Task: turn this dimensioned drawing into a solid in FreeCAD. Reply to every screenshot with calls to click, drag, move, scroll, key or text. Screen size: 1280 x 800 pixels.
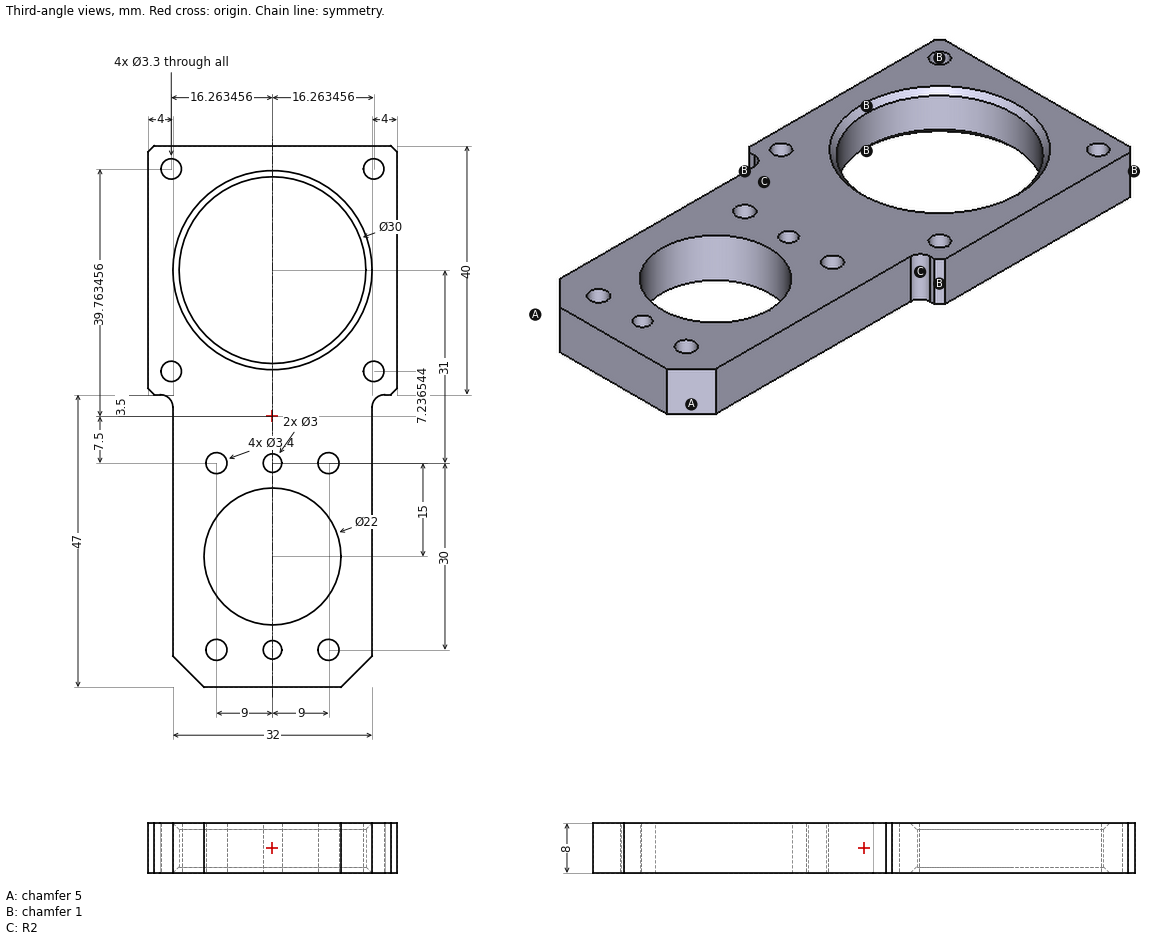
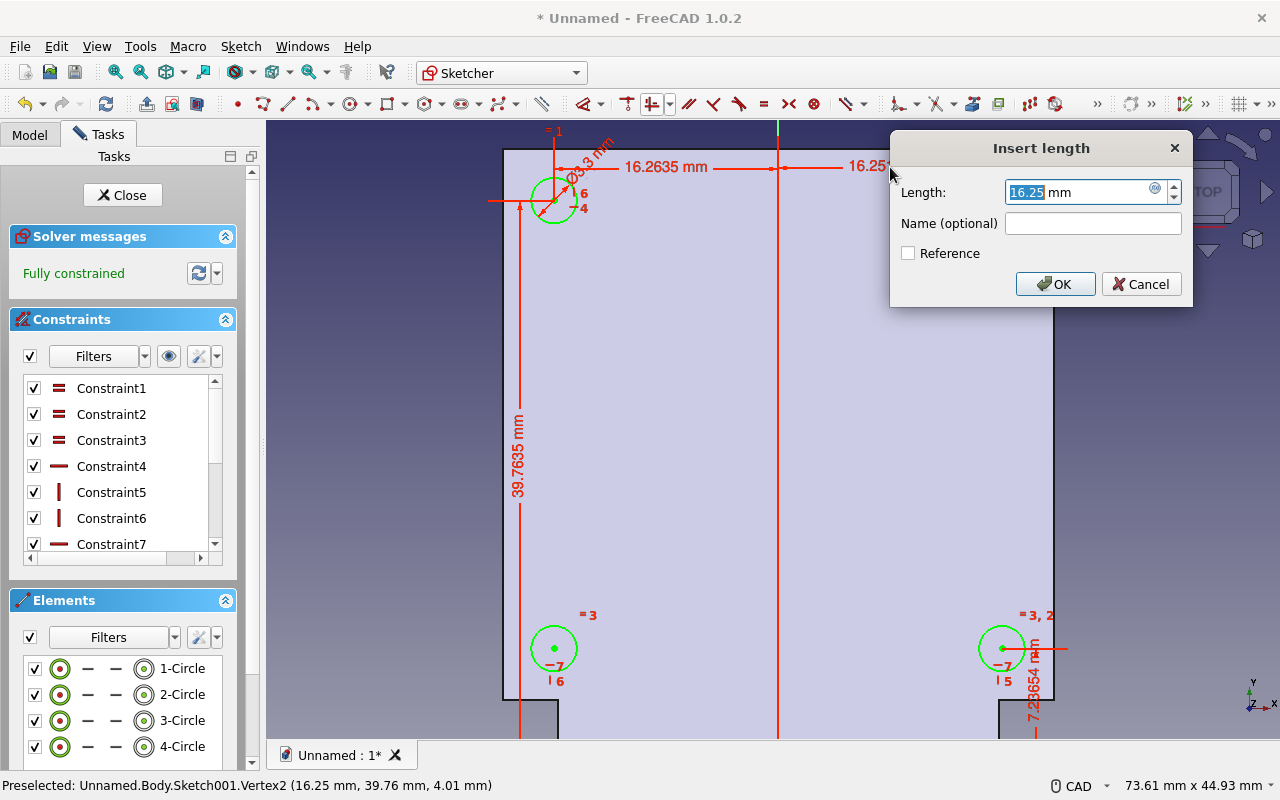
text(16.263456)
key(Return)
key(Escape)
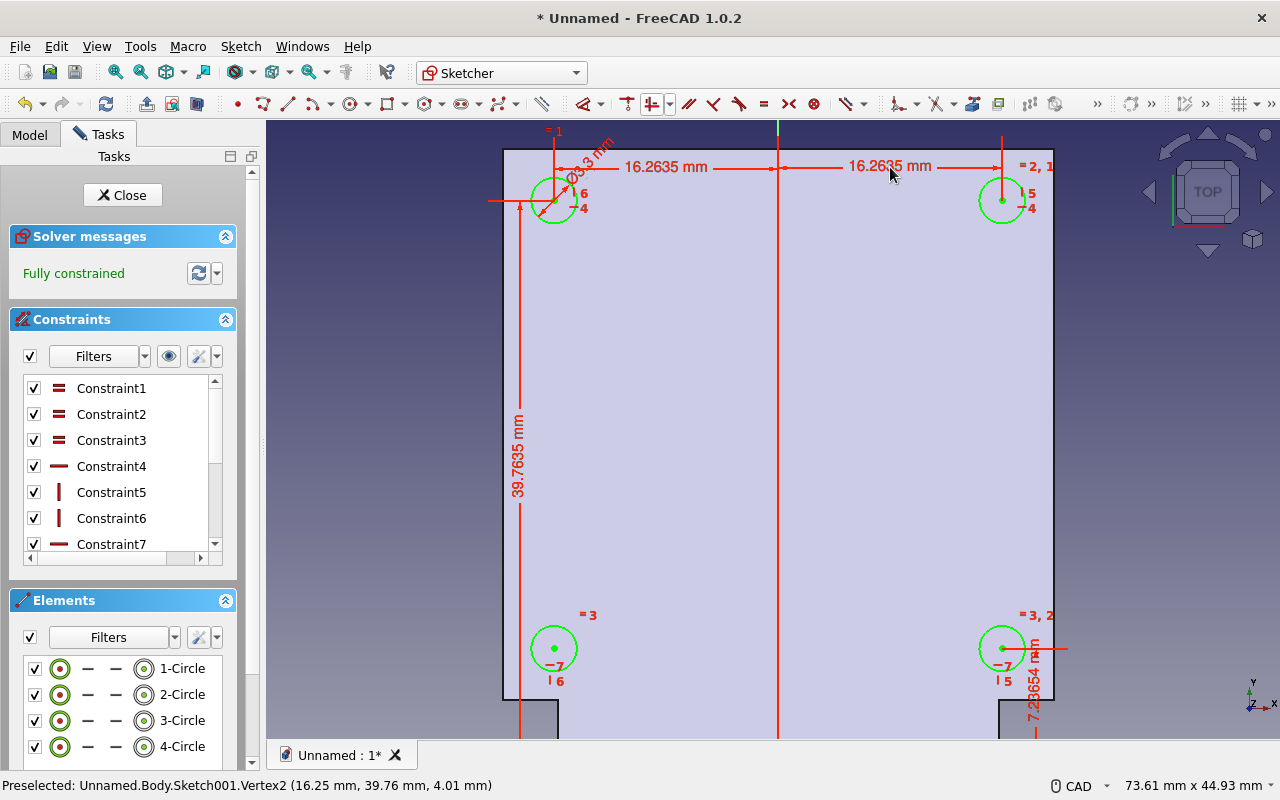
click(123, 195)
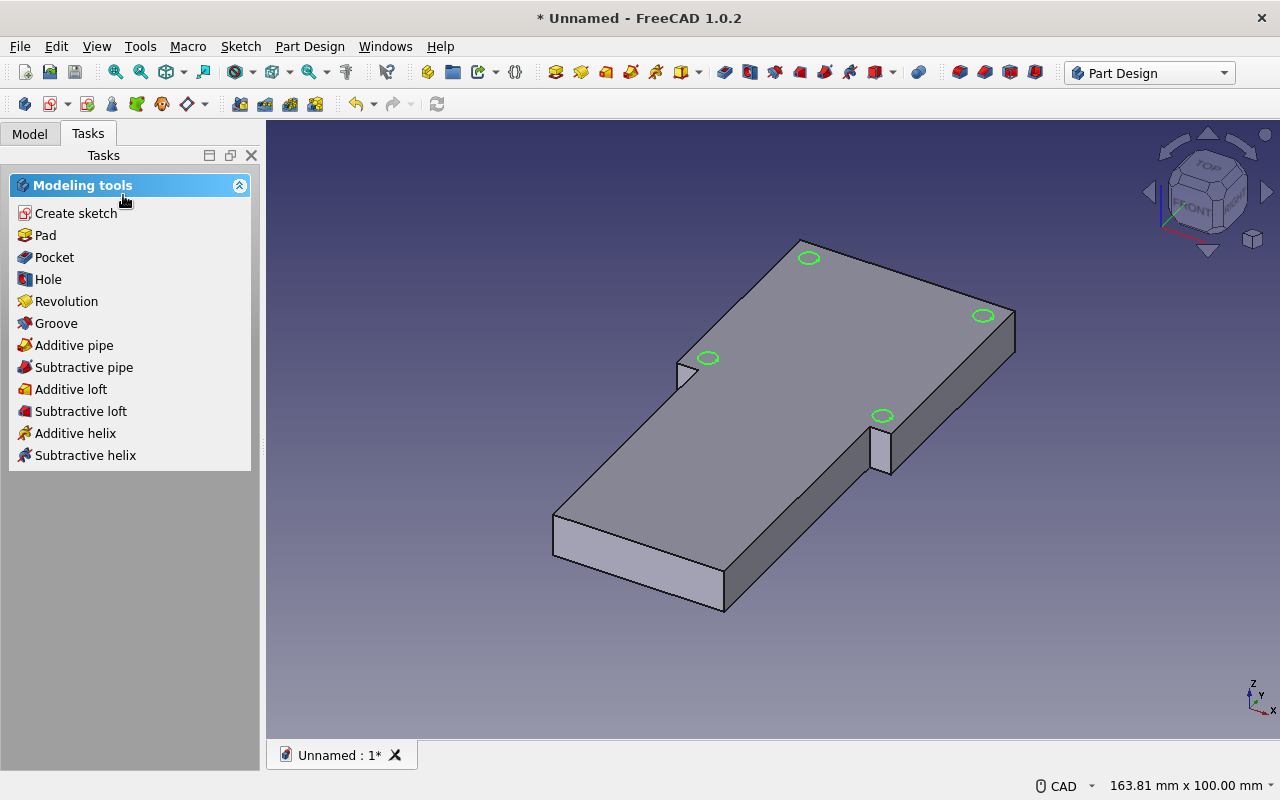
click(750, 72)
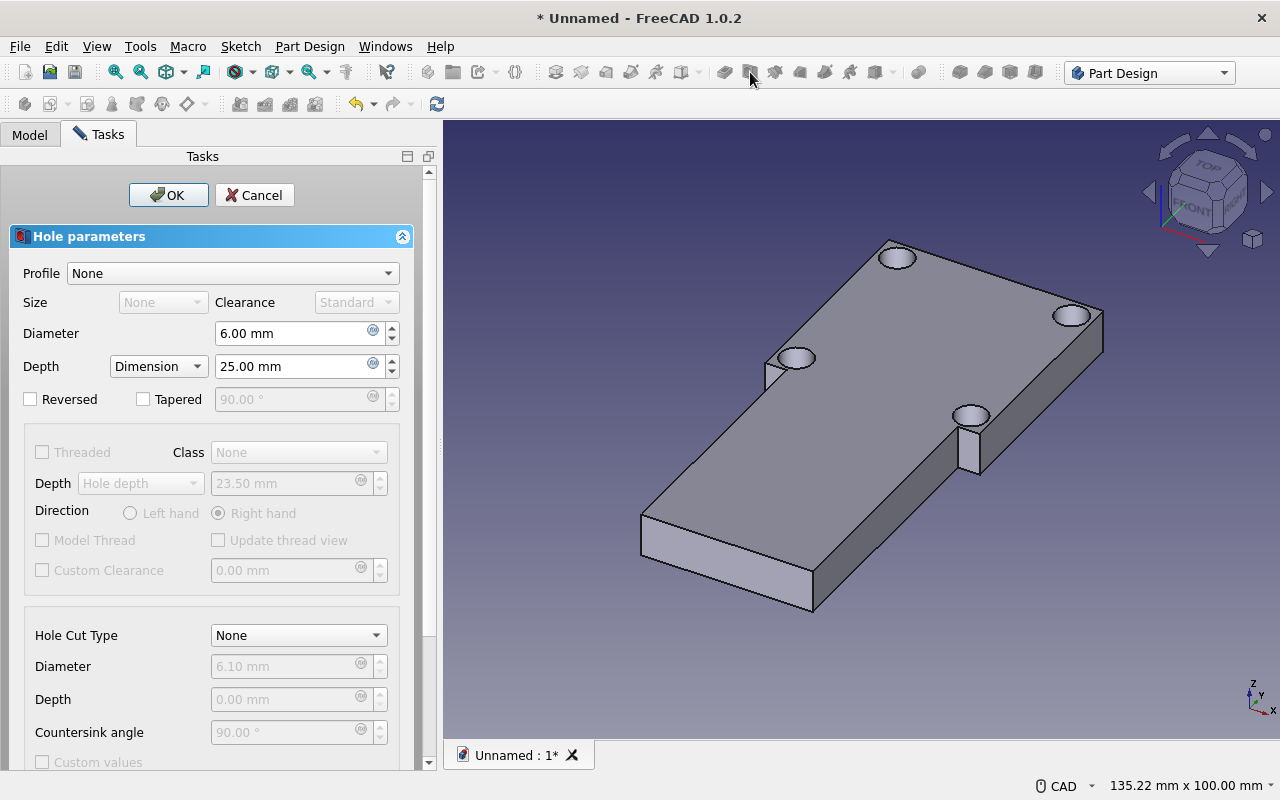
triple_click(300, 334)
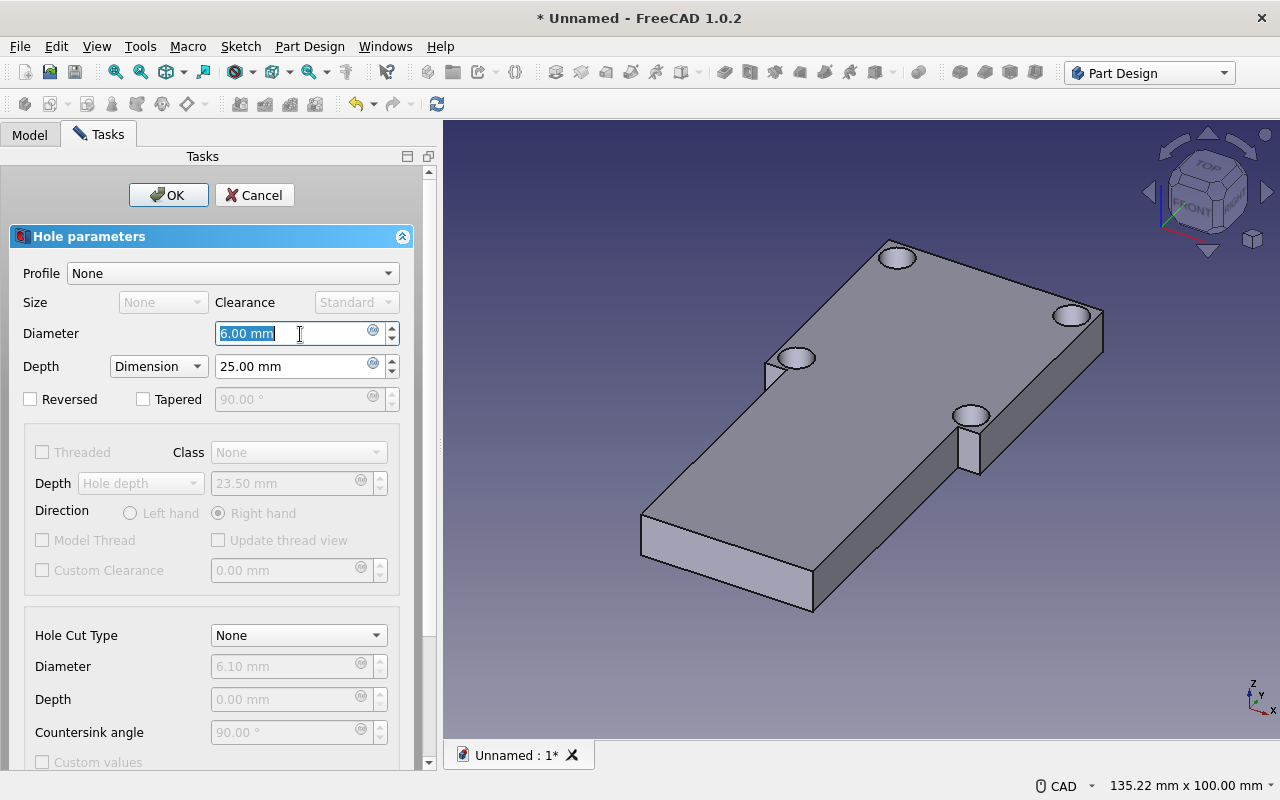
text(3.3)
key(Tab)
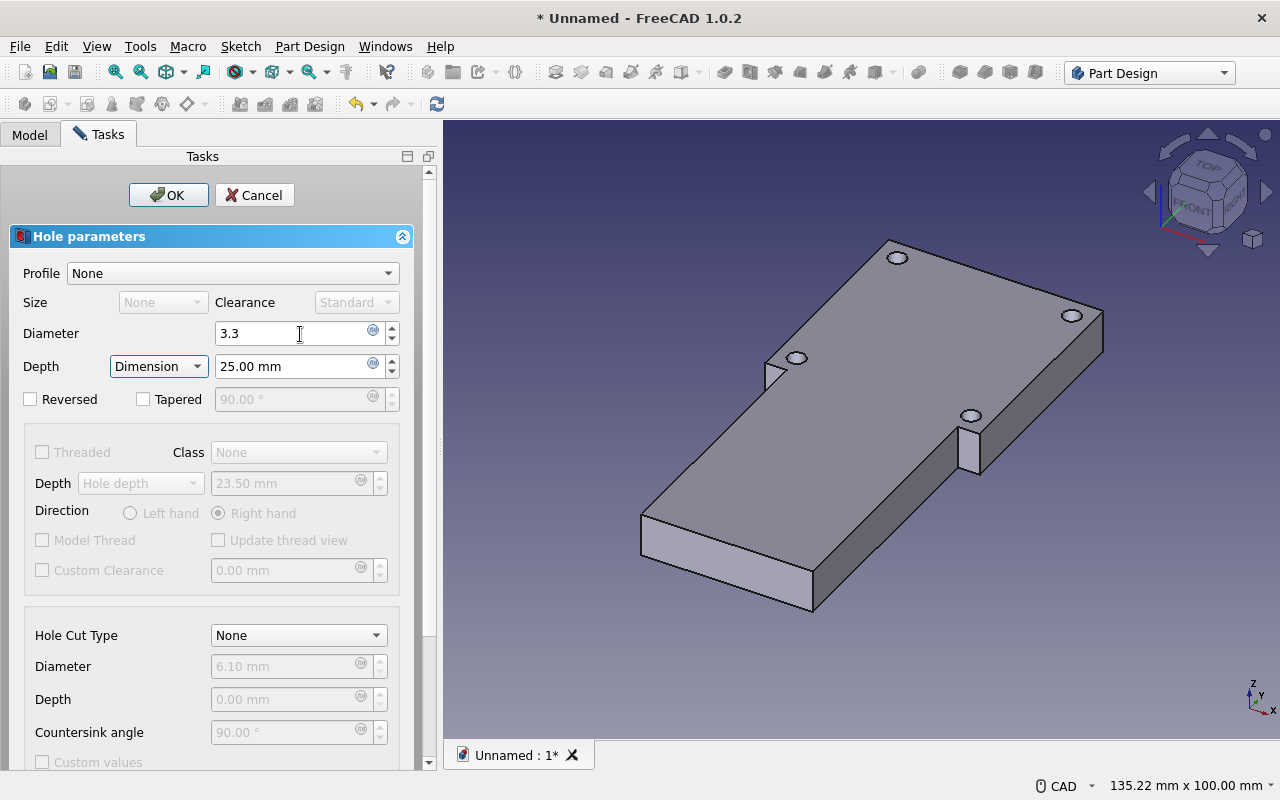
click(160, 366)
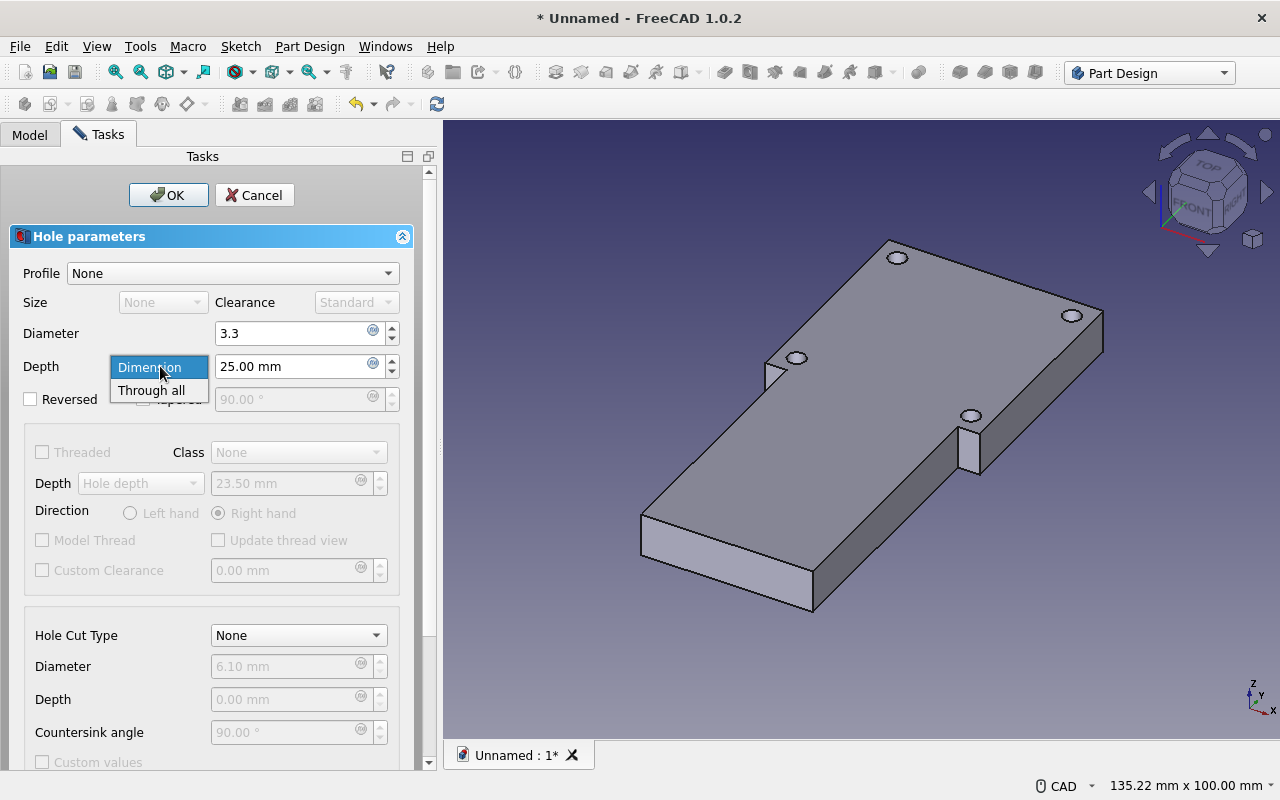
click(158, 390)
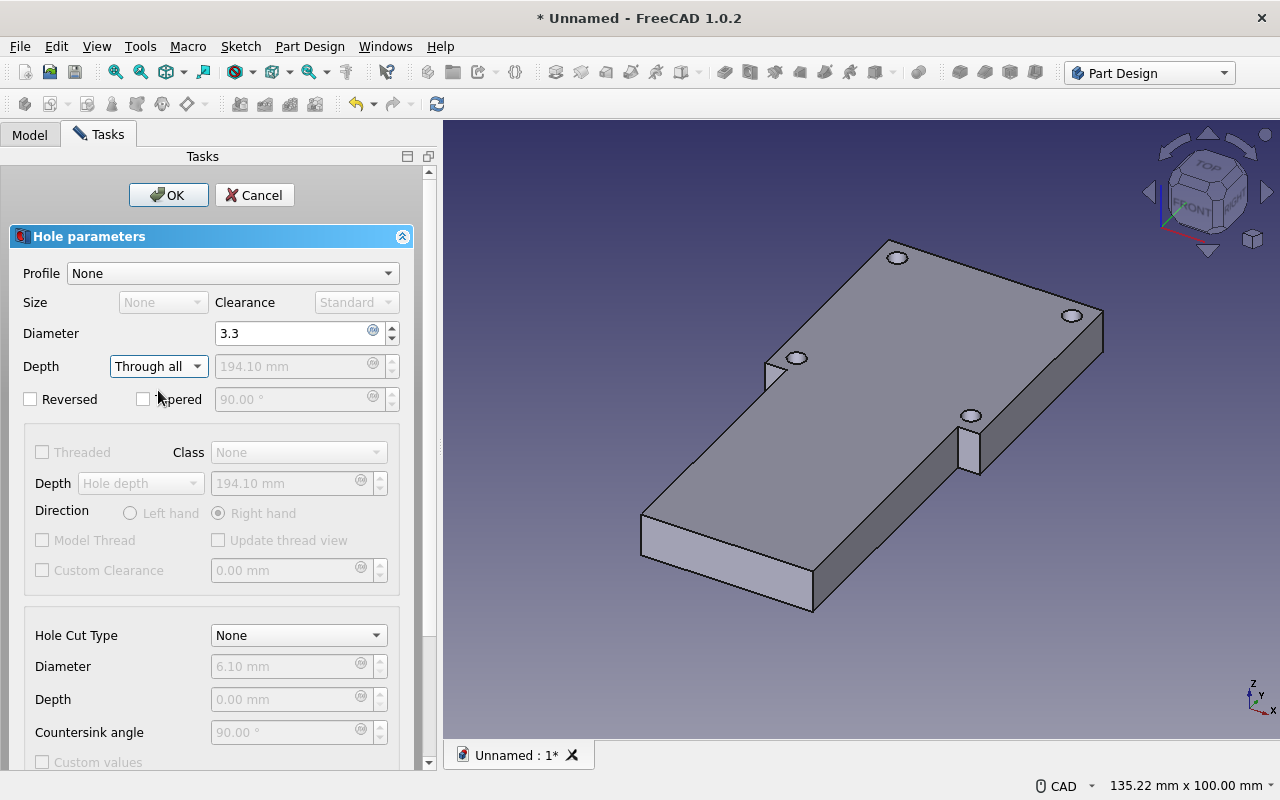
click(169, 195)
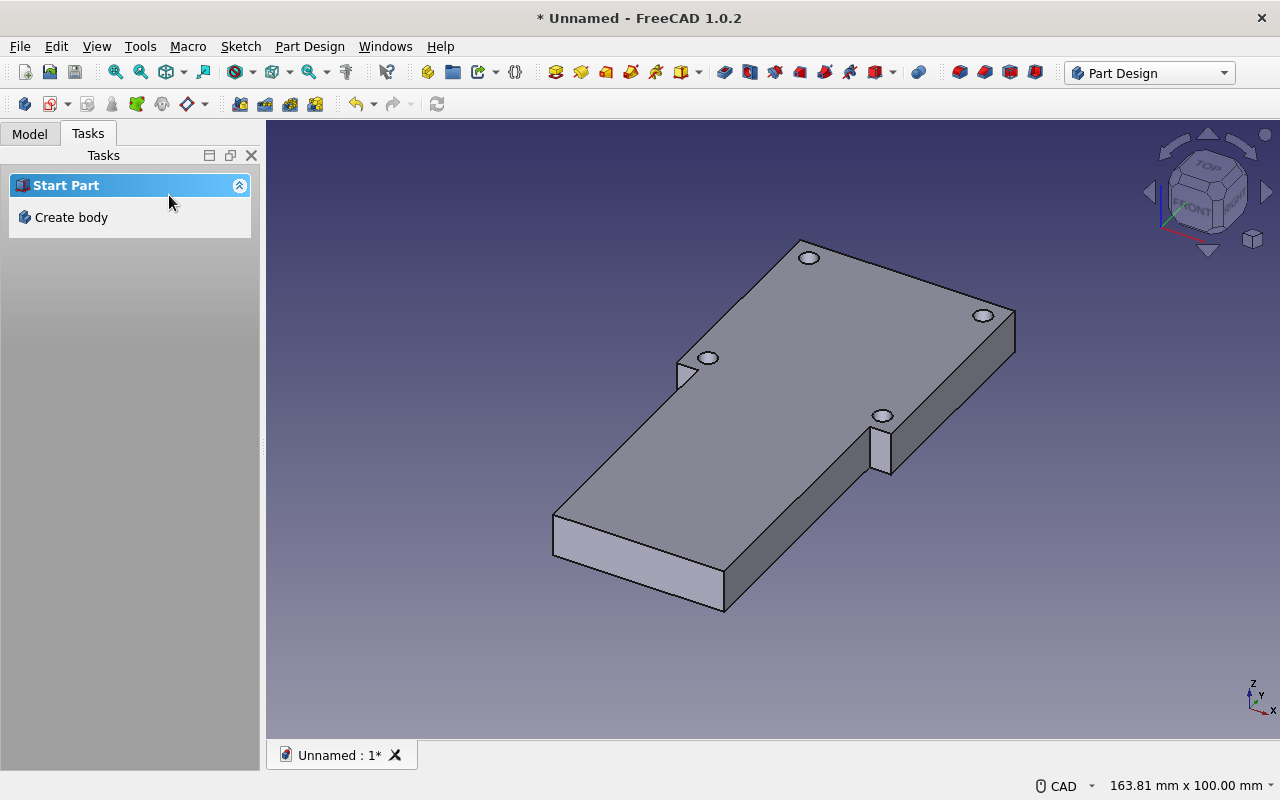
click(850, 332)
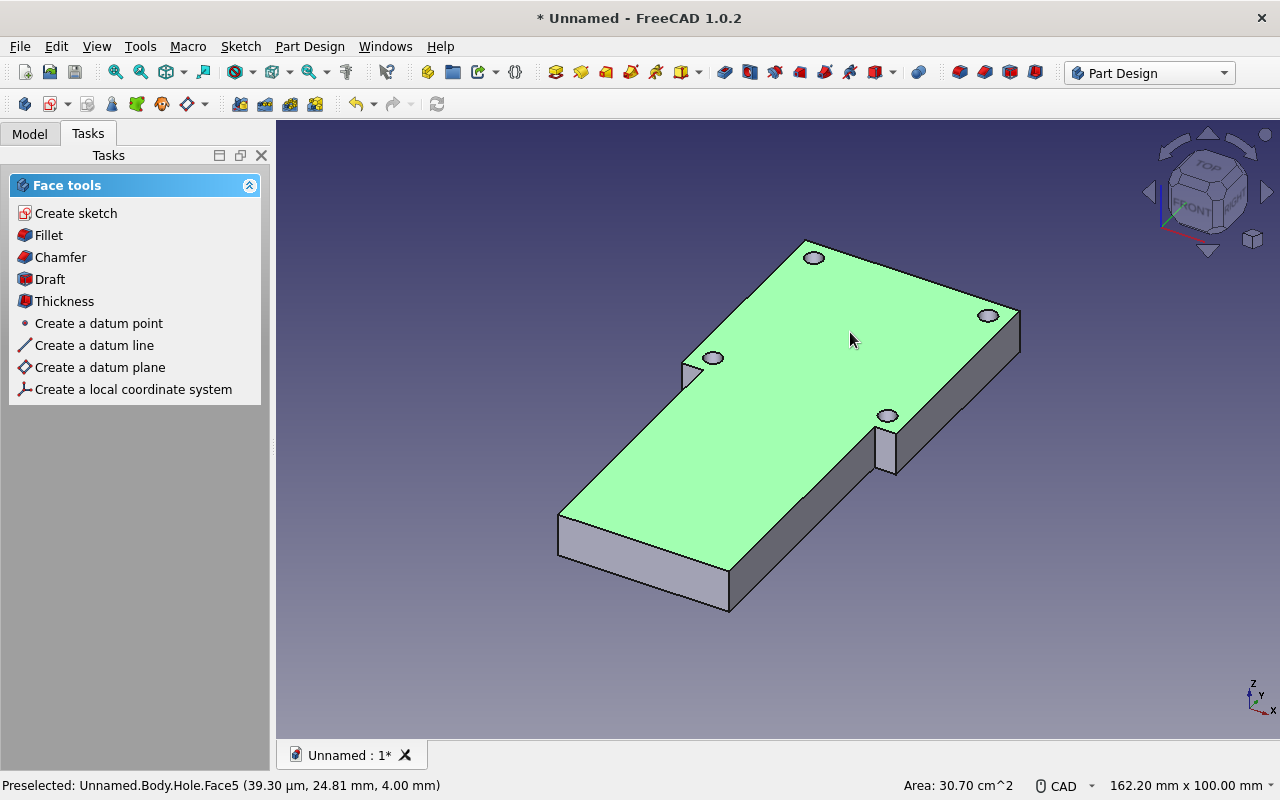
click(50, 104)